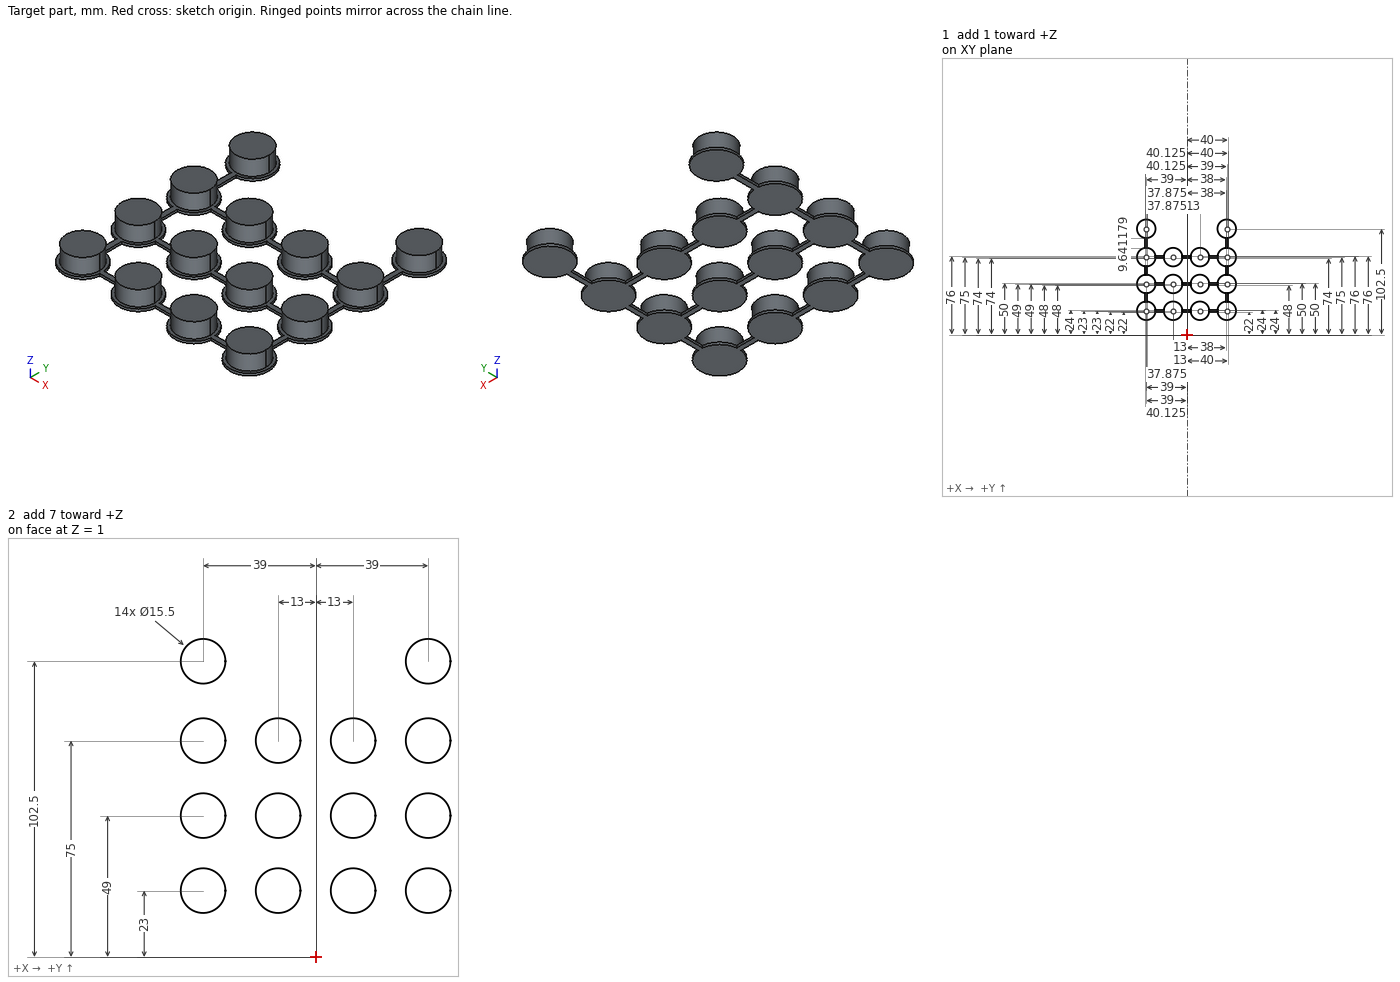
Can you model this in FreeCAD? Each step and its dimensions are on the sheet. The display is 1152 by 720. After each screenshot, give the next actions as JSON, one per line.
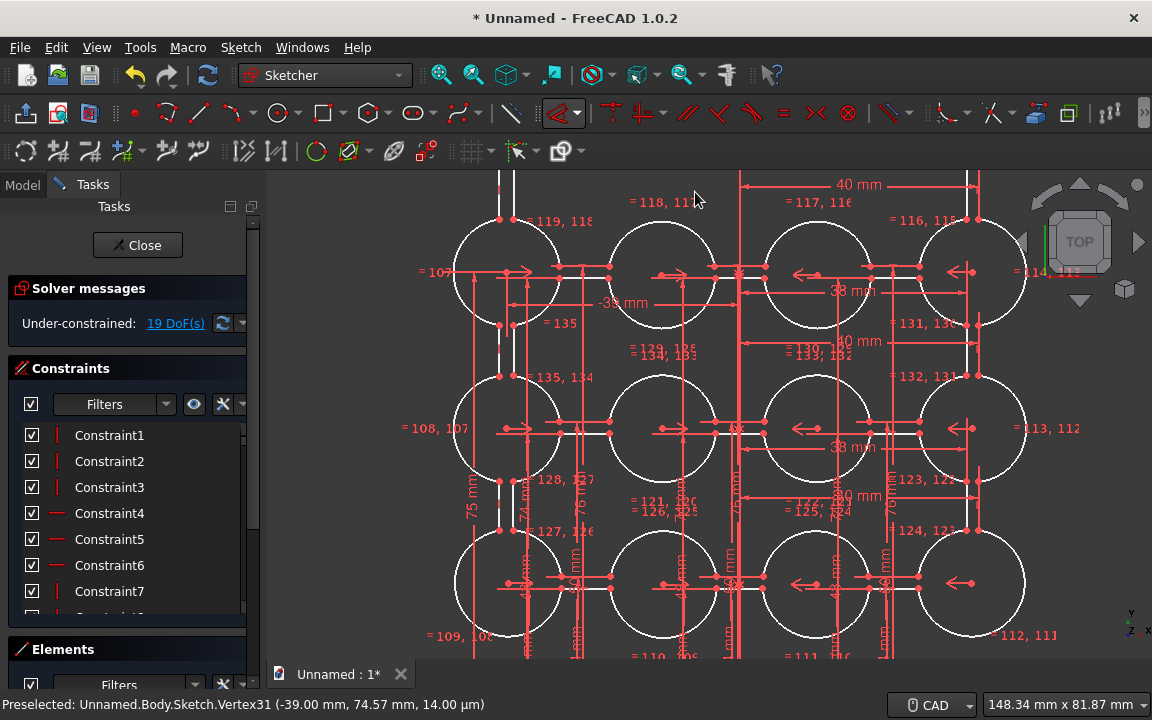
{"action": "left_click", "coordinate": [507, 429]}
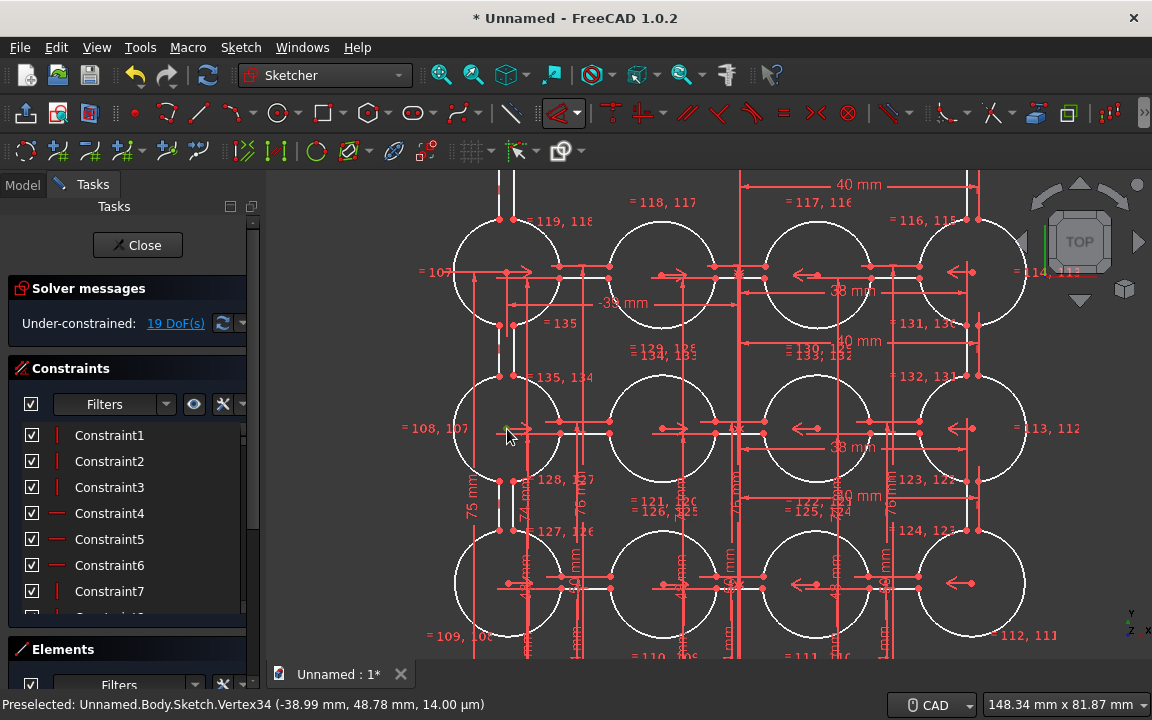
{"action": "key", "text": "l"}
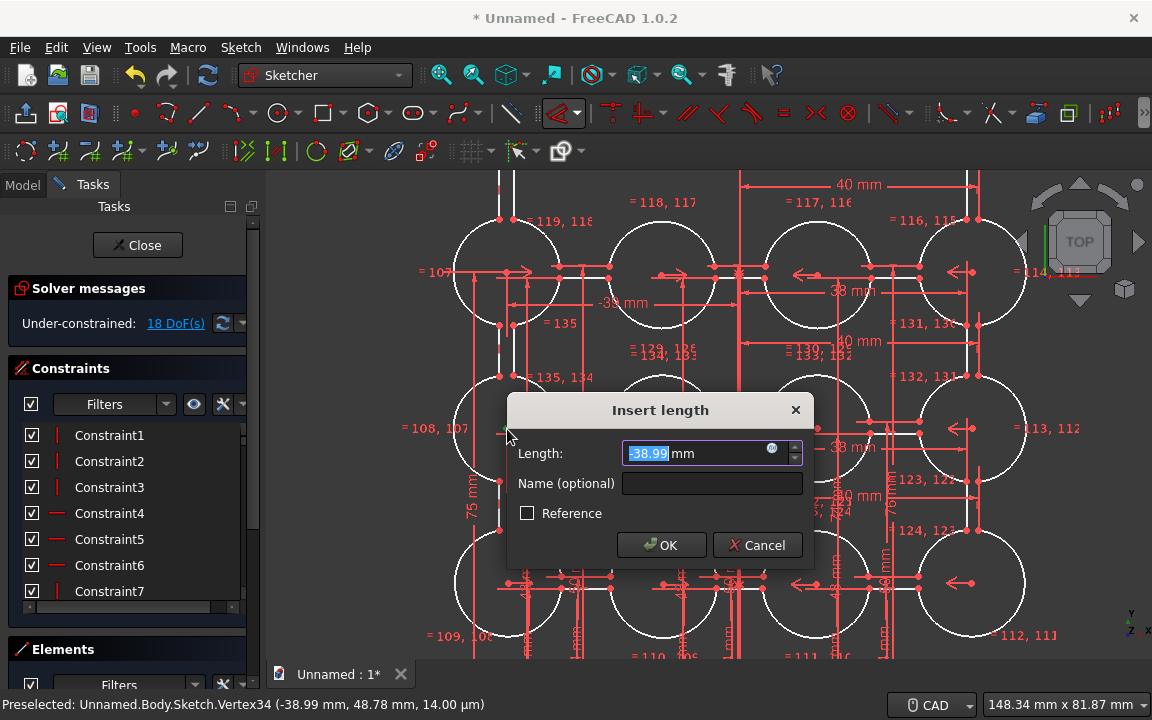
{"action": "type", "text": "-39"}
{"action": "key", "text": "Return"}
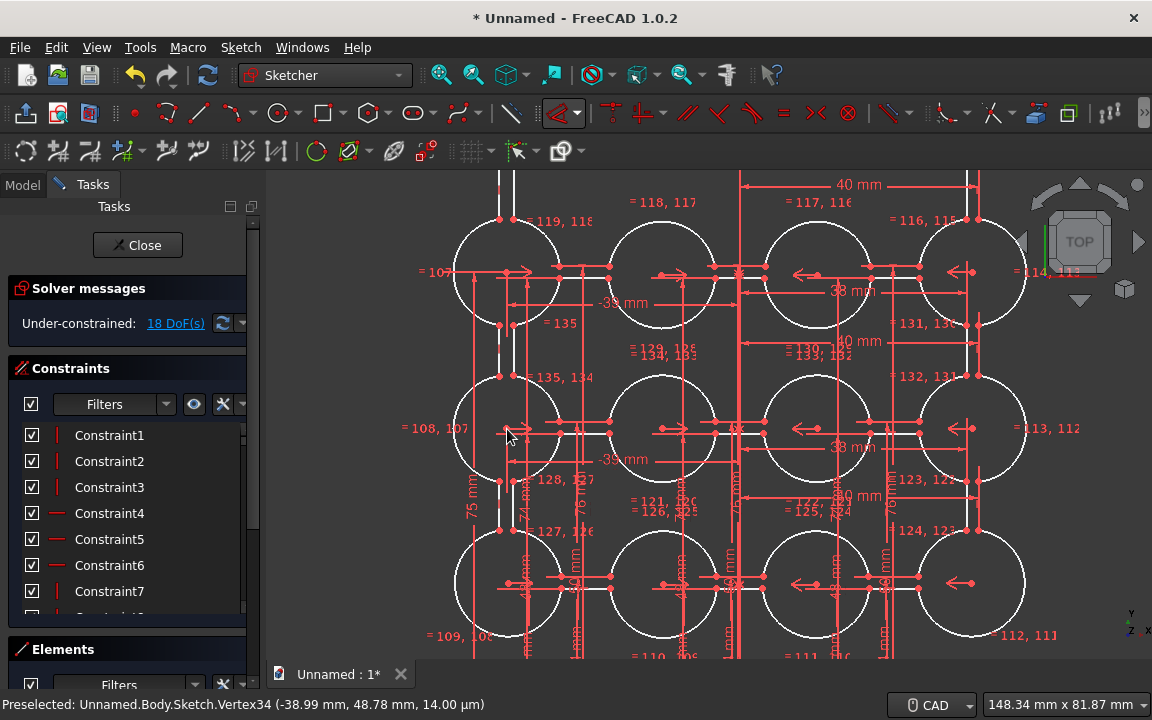
{"action": "left_click", "coordinate": [507, 429]}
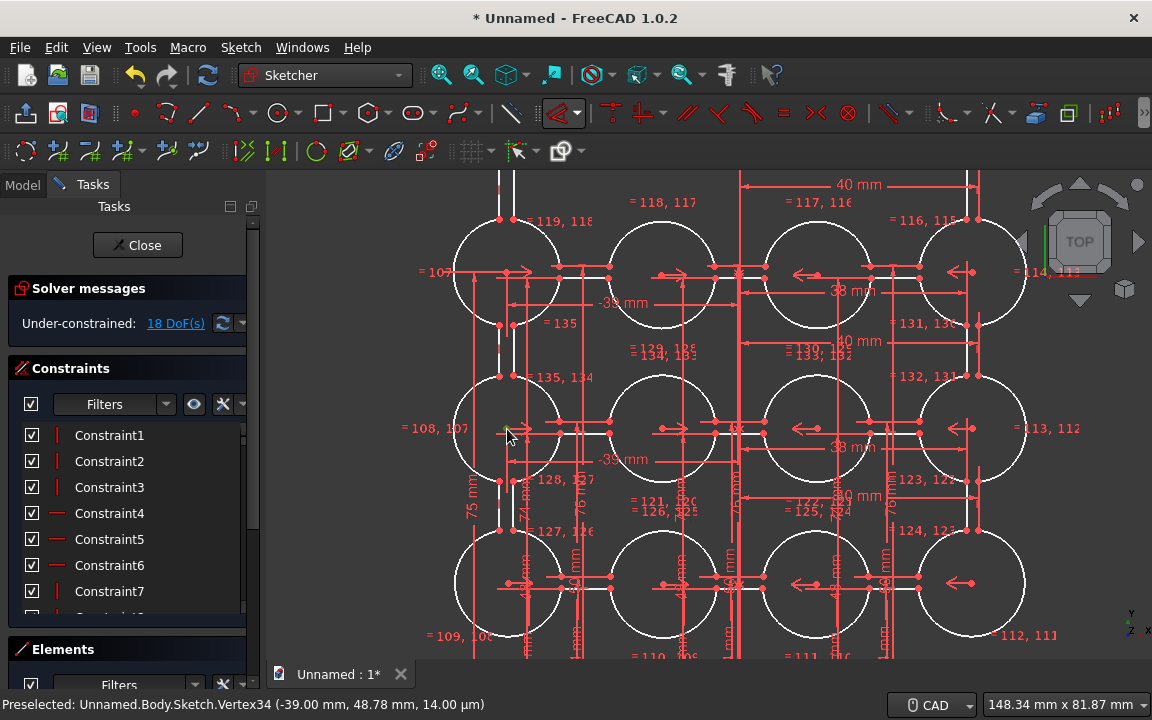
{"action": "left_click", "coordinate": [580, 114]}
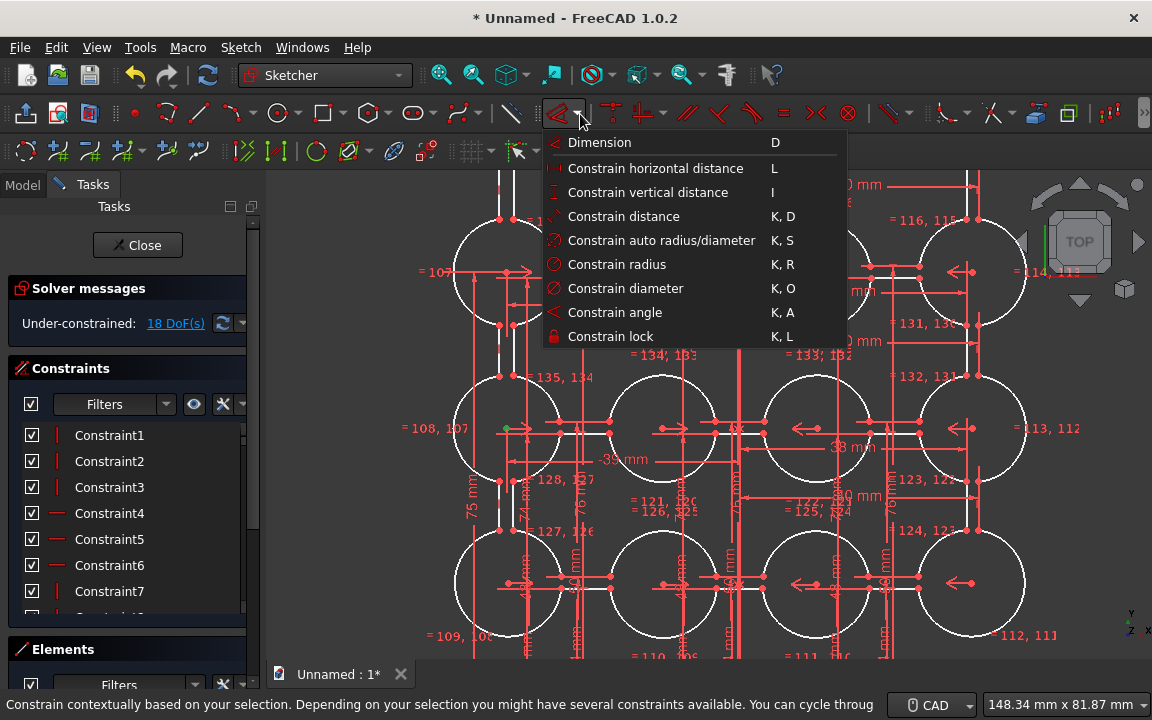
{"action": "left_click", "coordinate": [695, 192]}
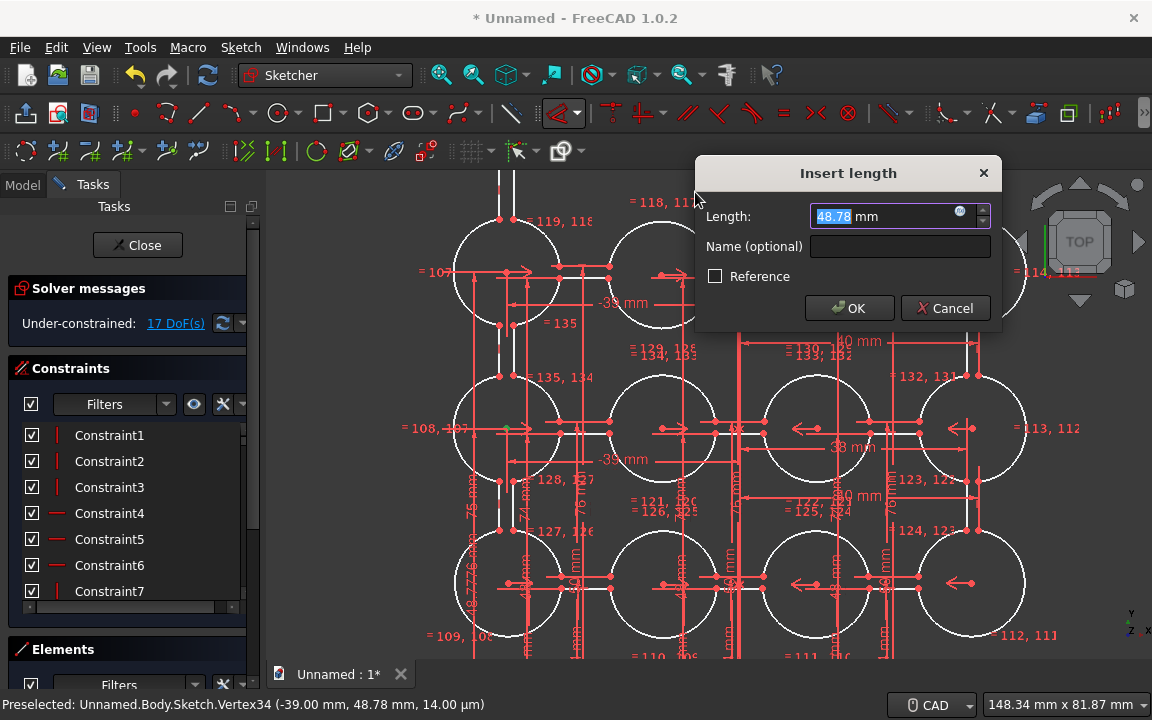
{"action": "type", "text": "49"}
{"action": "key", "text": "Return"}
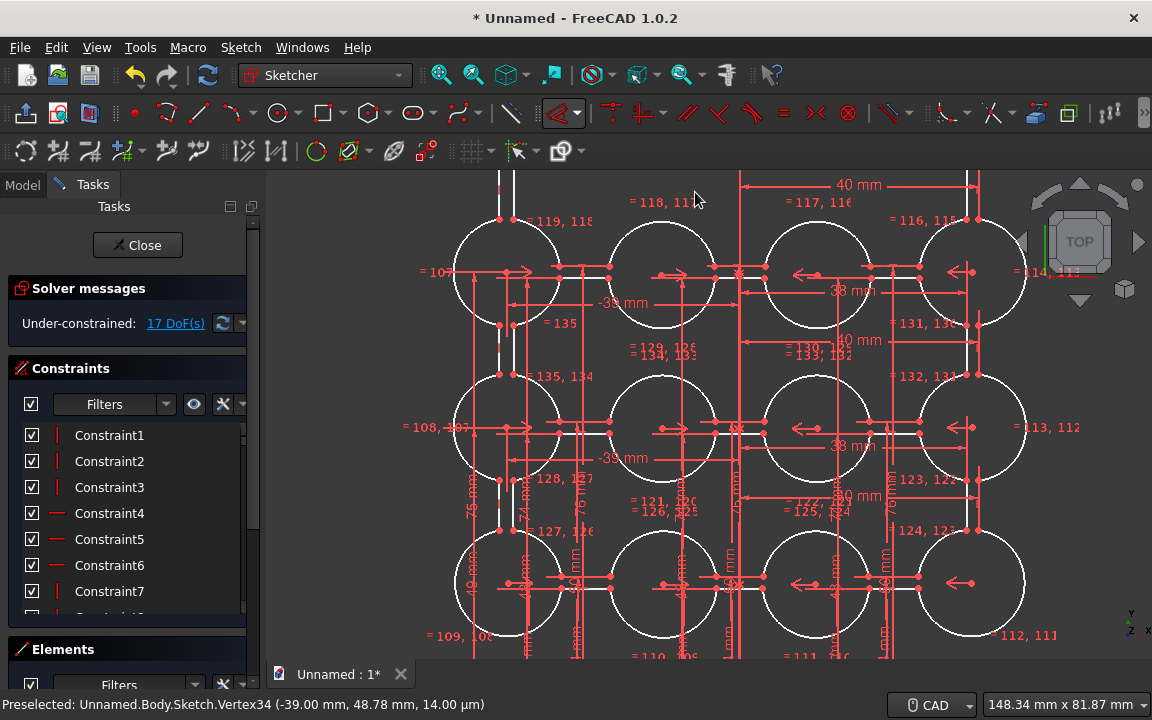
{"action": "left_click", "coordinate": [508, 583]}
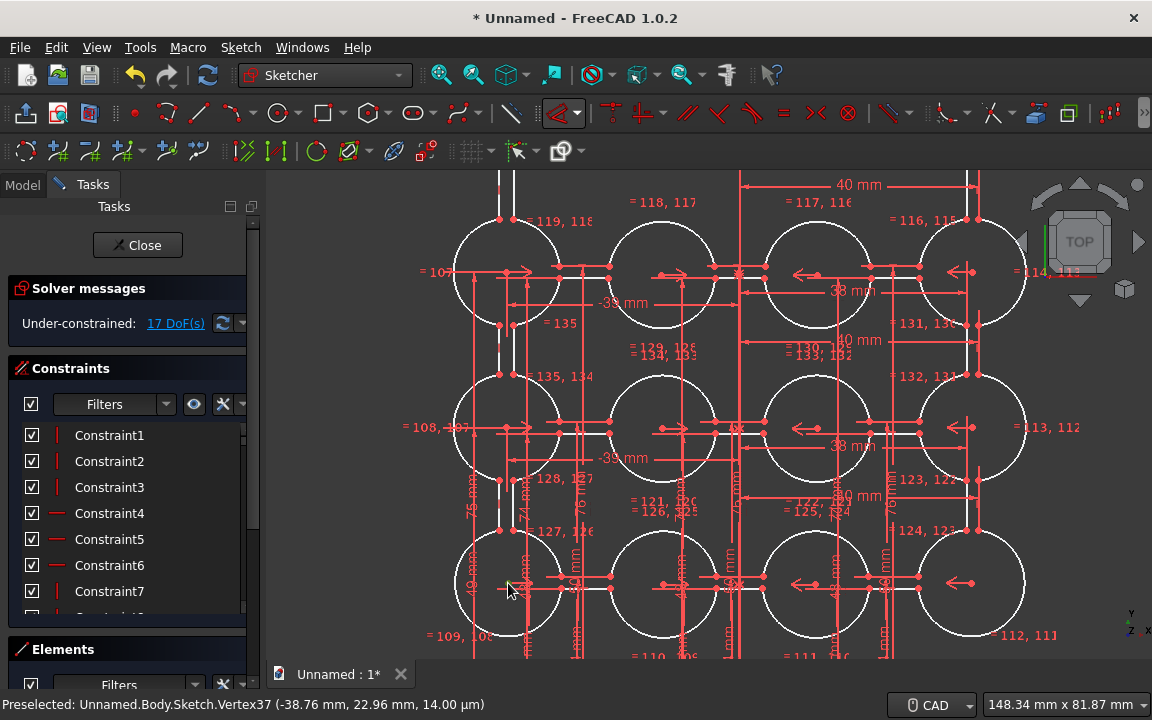
{"action": "left_click", "coordinate": [580, 114]}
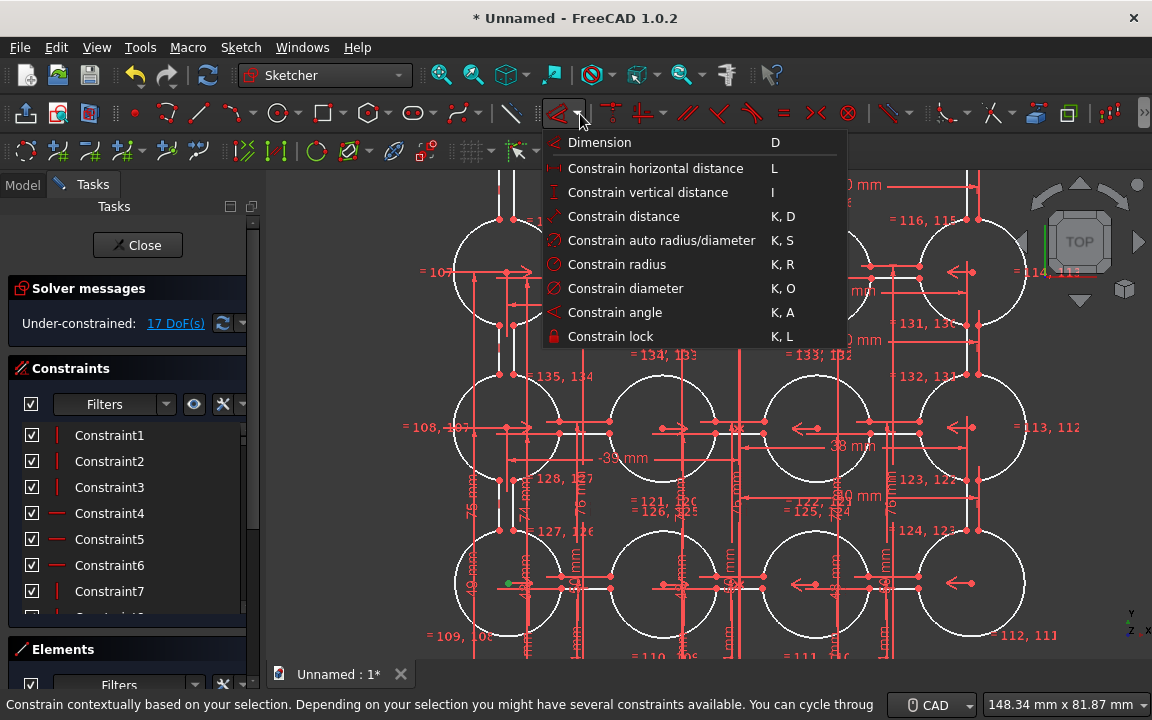
{"action": "left_click", "coordinate": [695, 168]}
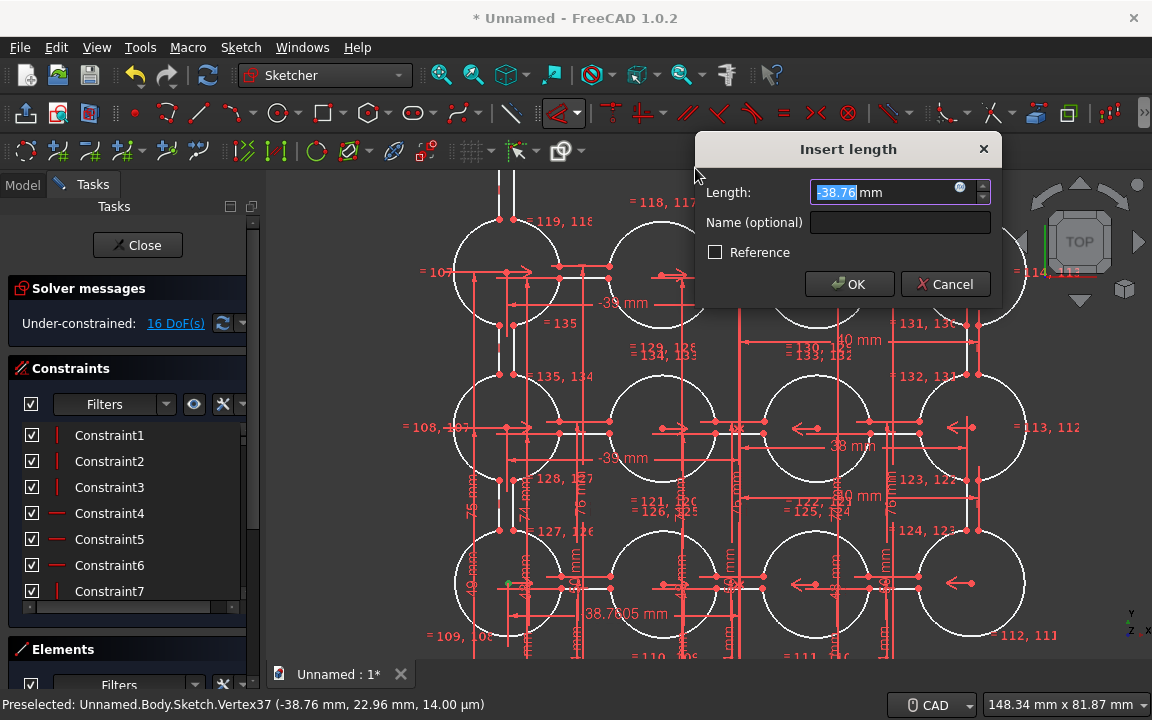
{"action": "type", "text": "-39"}
{"action": "key", "text": "Return"}